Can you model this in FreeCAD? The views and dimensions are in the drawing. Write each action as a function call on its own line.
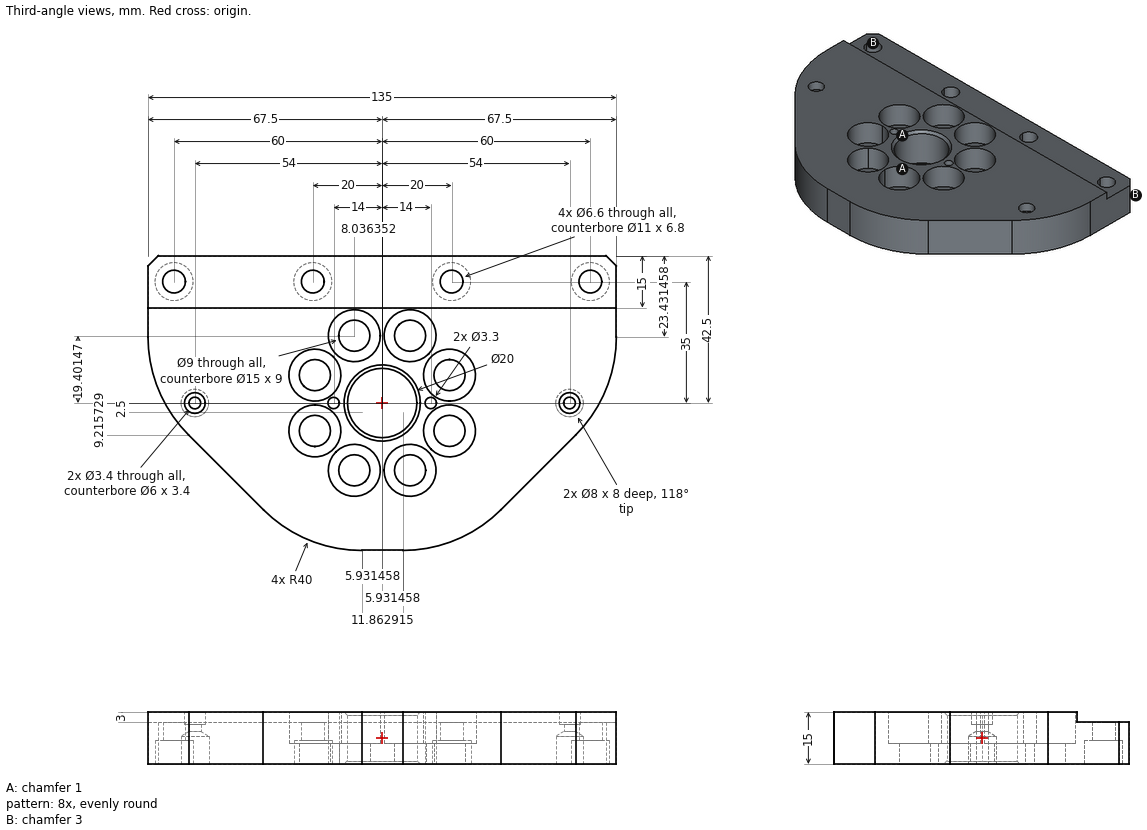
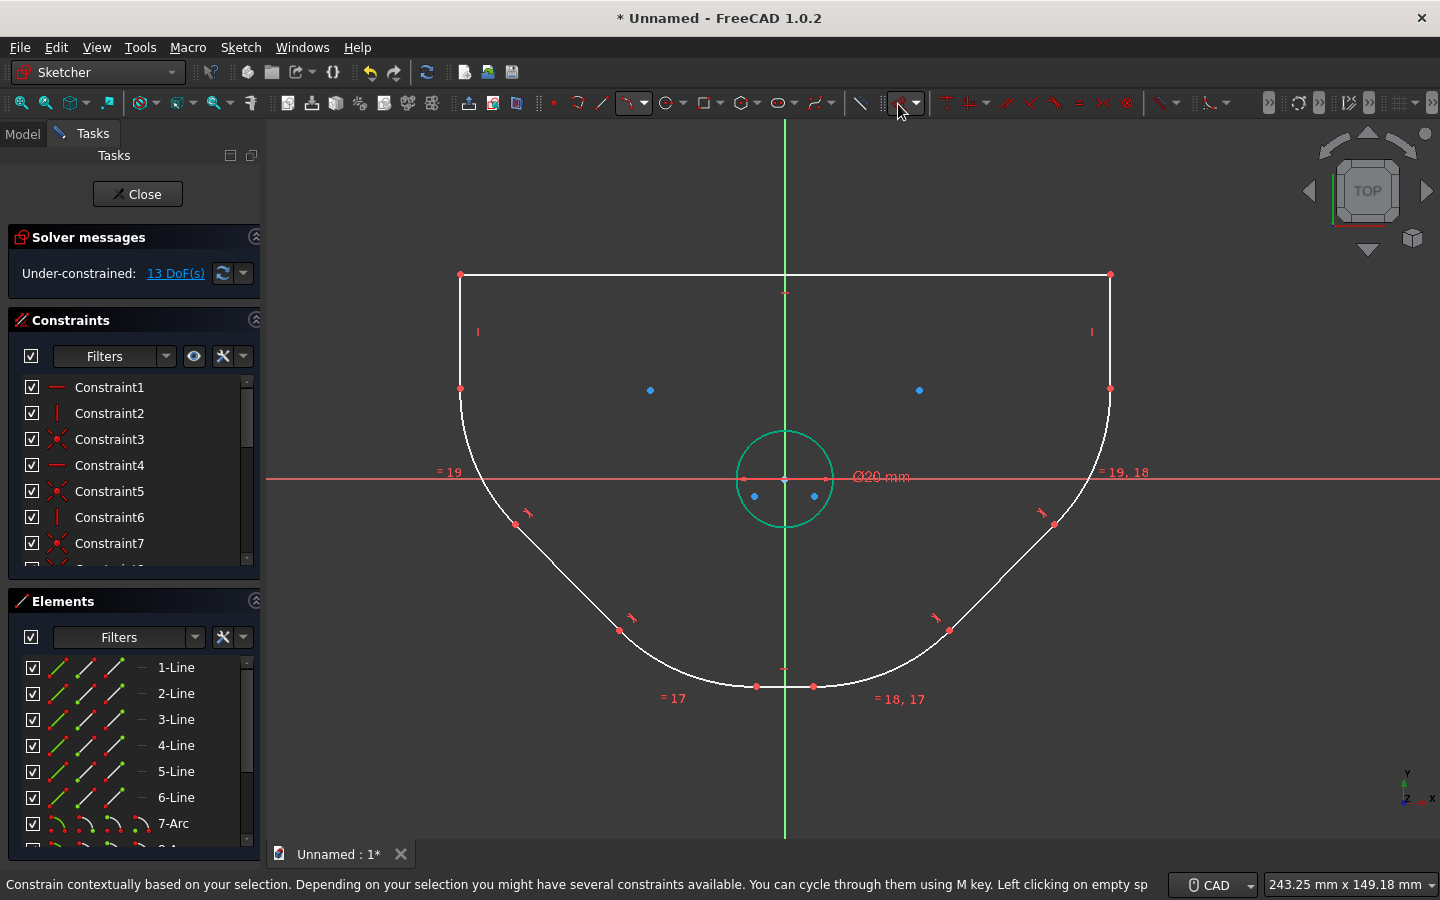
click(655, 659)
click(638, 686)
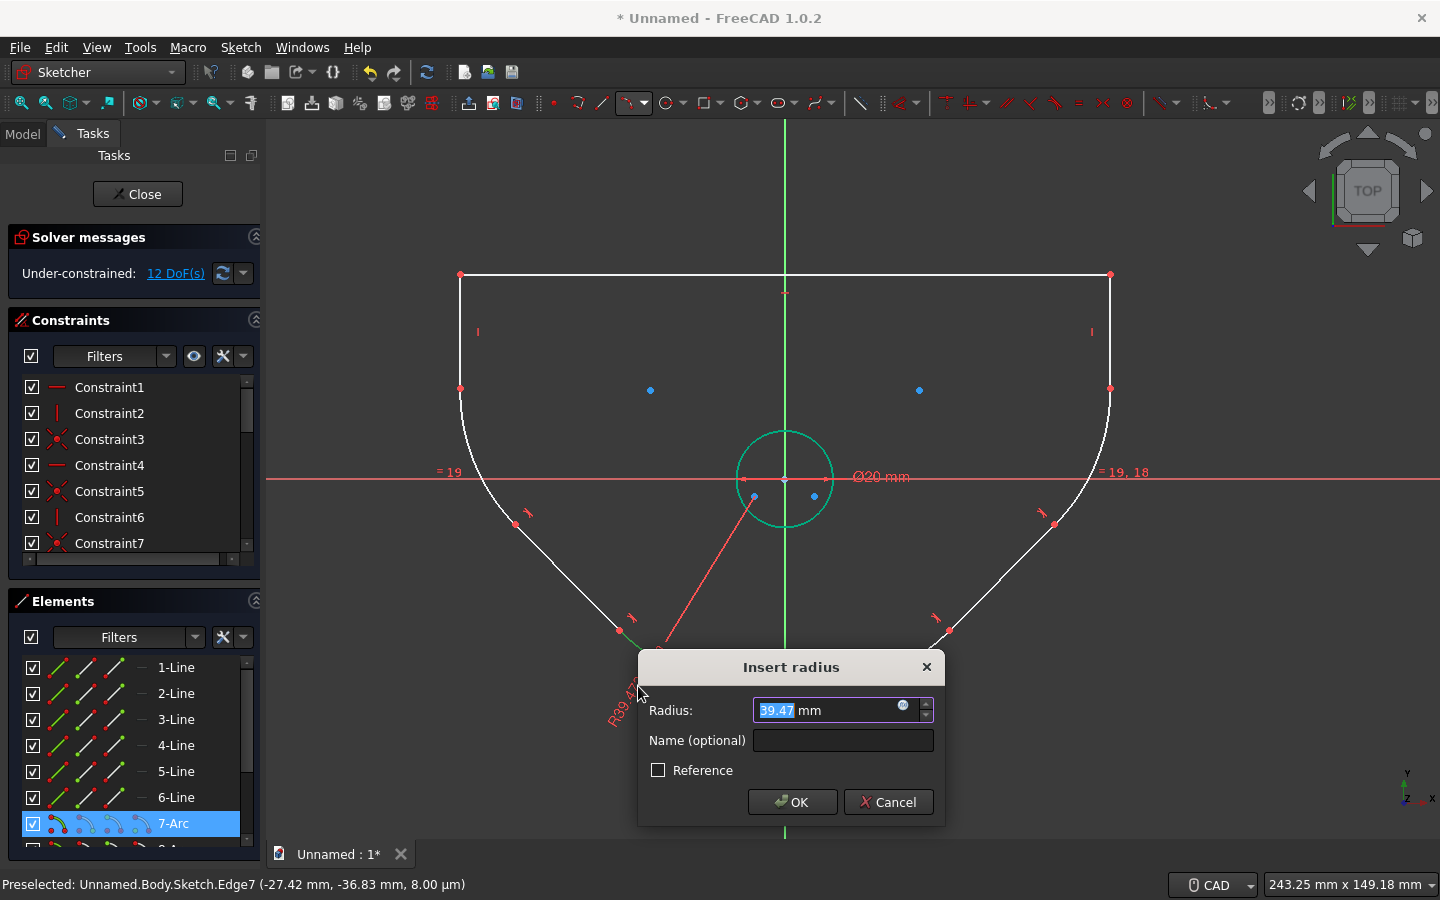
text(40)
key(Return)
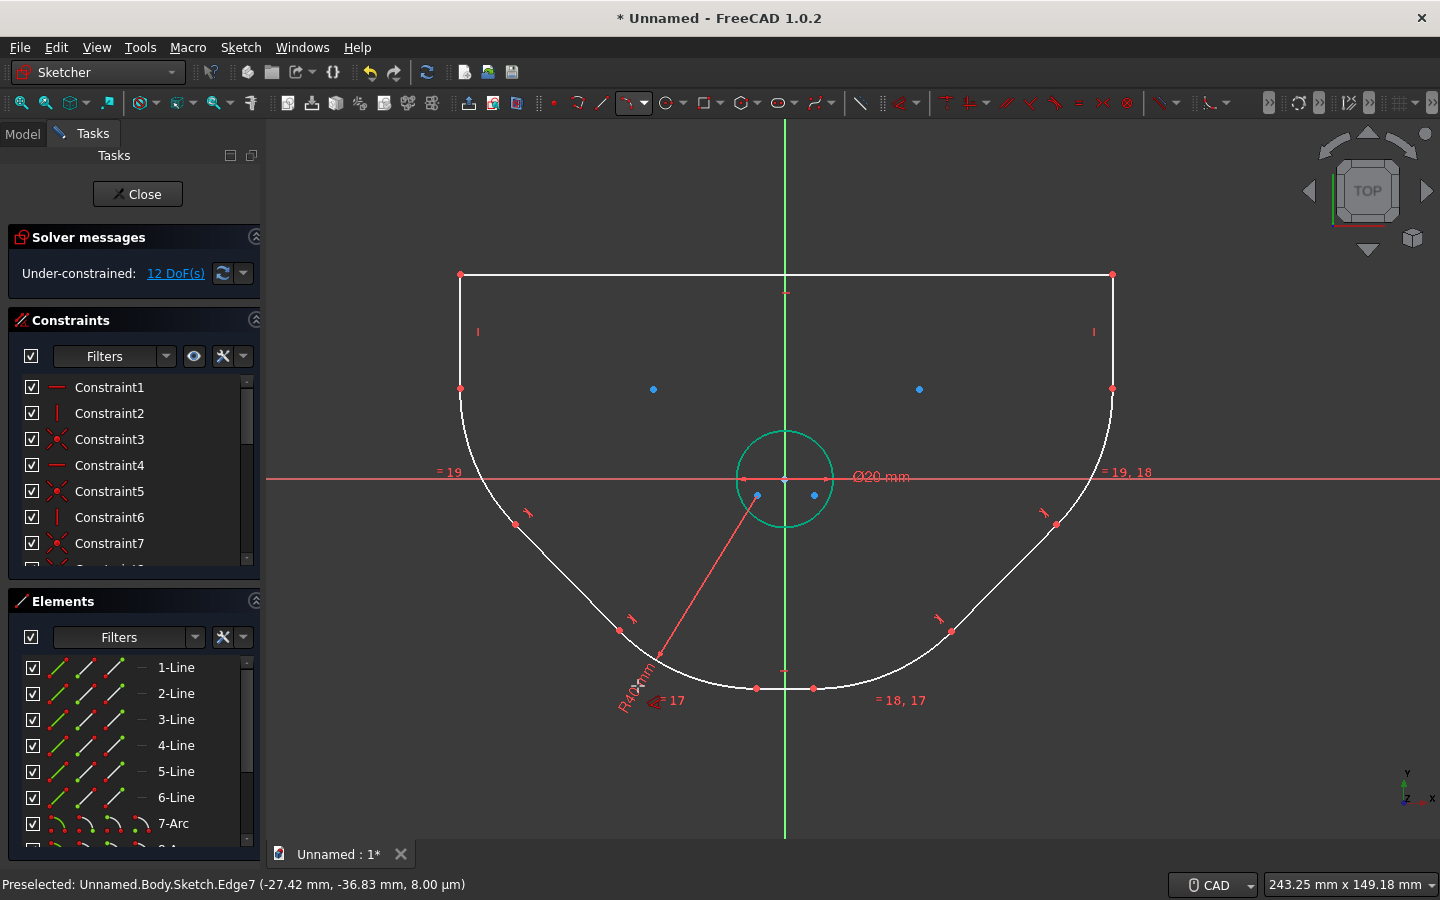
click(917, 275)
click(636, 241)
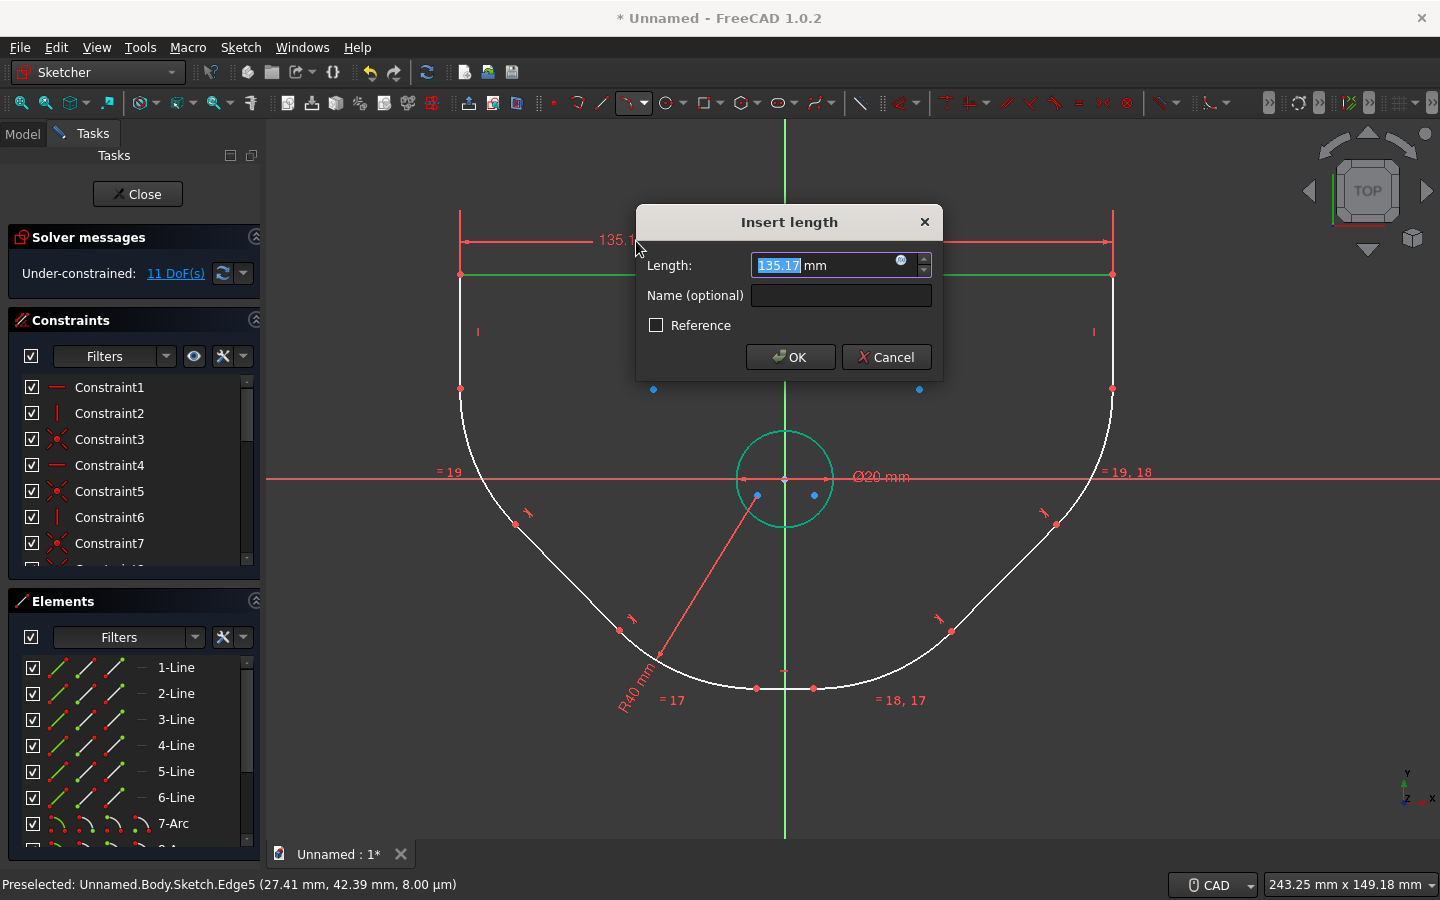
text(135)
key(Return)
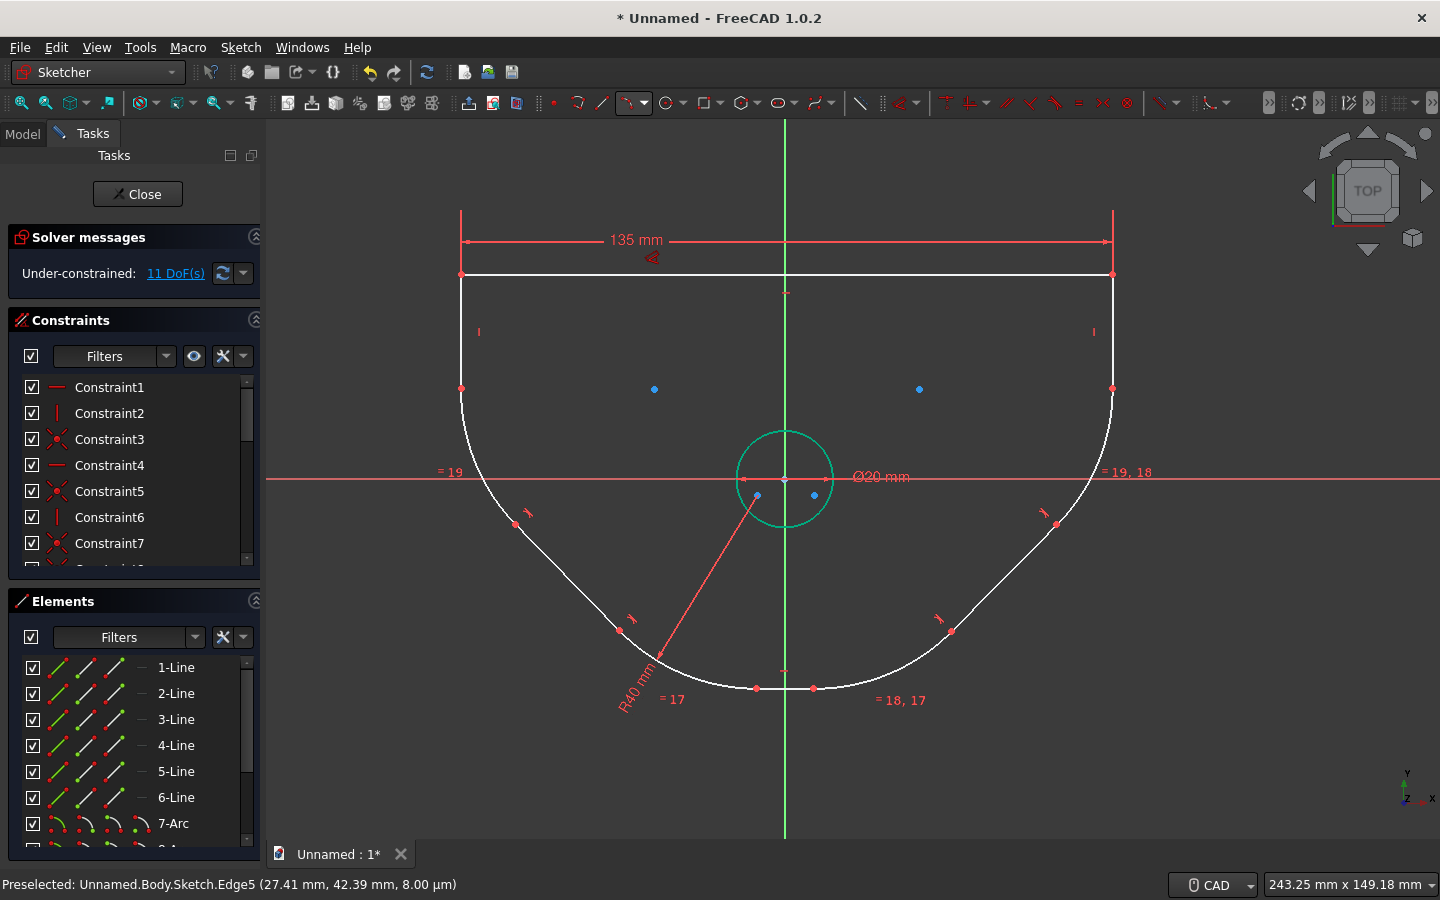
scroll(757, 496, up, 6)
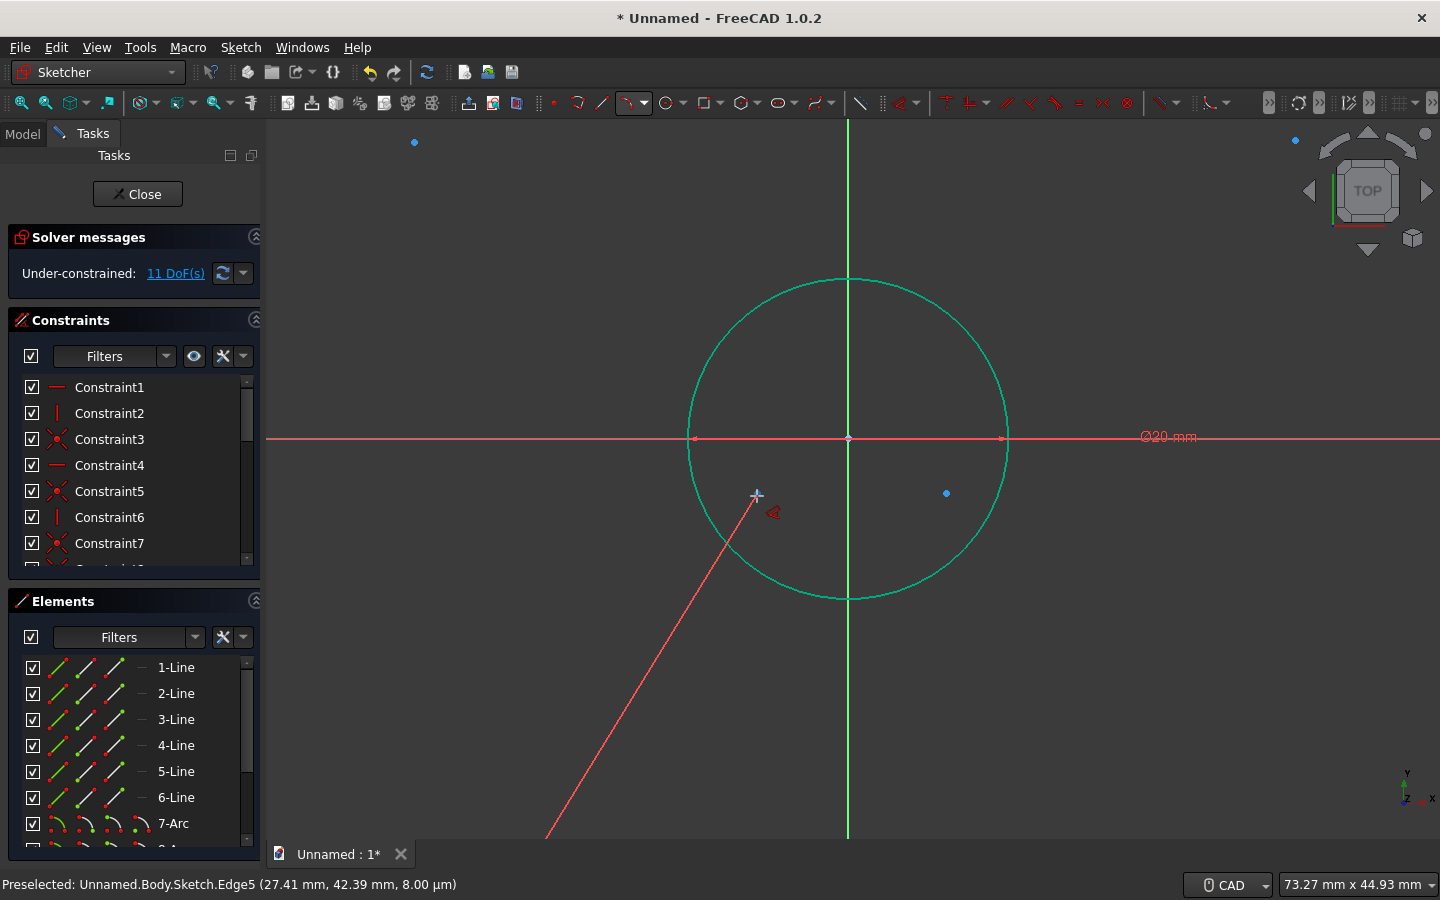
click(757, 494)
click(723, 466)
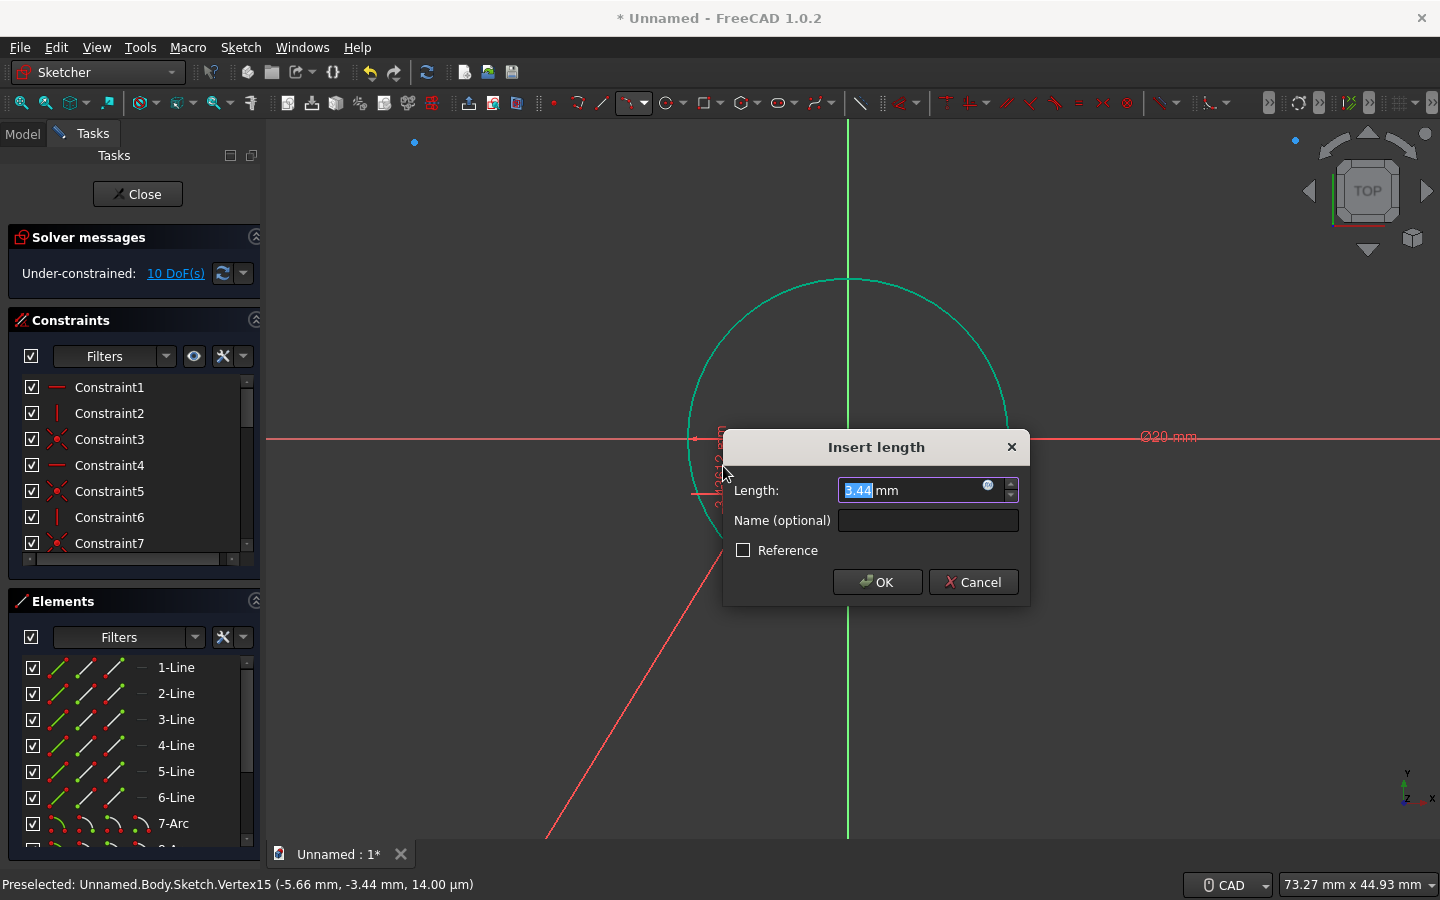
text(2.5)
key(Return)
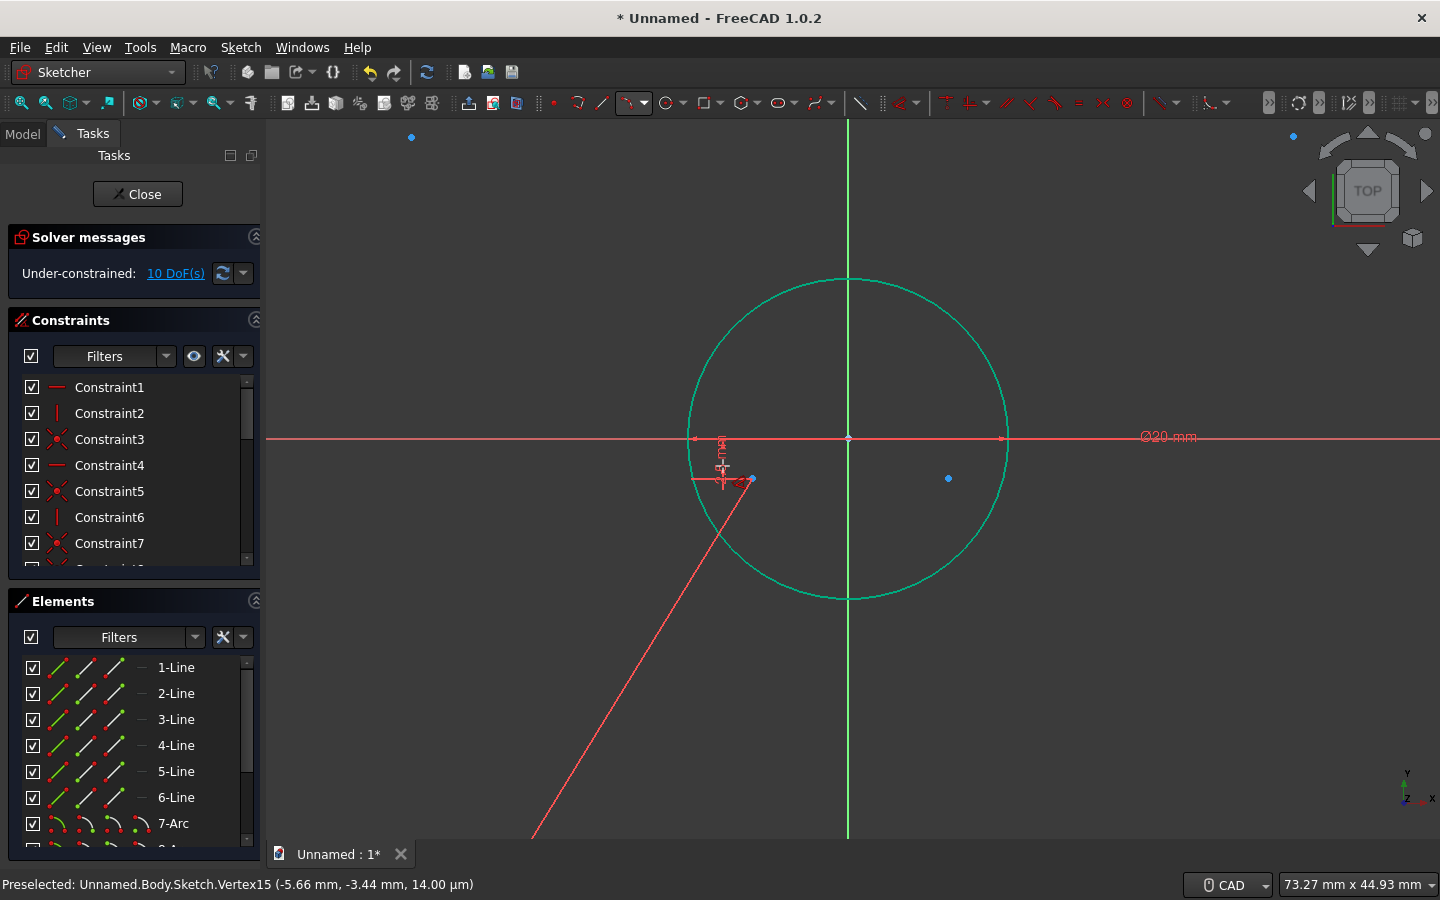
scroll(757, 496, down, 6)